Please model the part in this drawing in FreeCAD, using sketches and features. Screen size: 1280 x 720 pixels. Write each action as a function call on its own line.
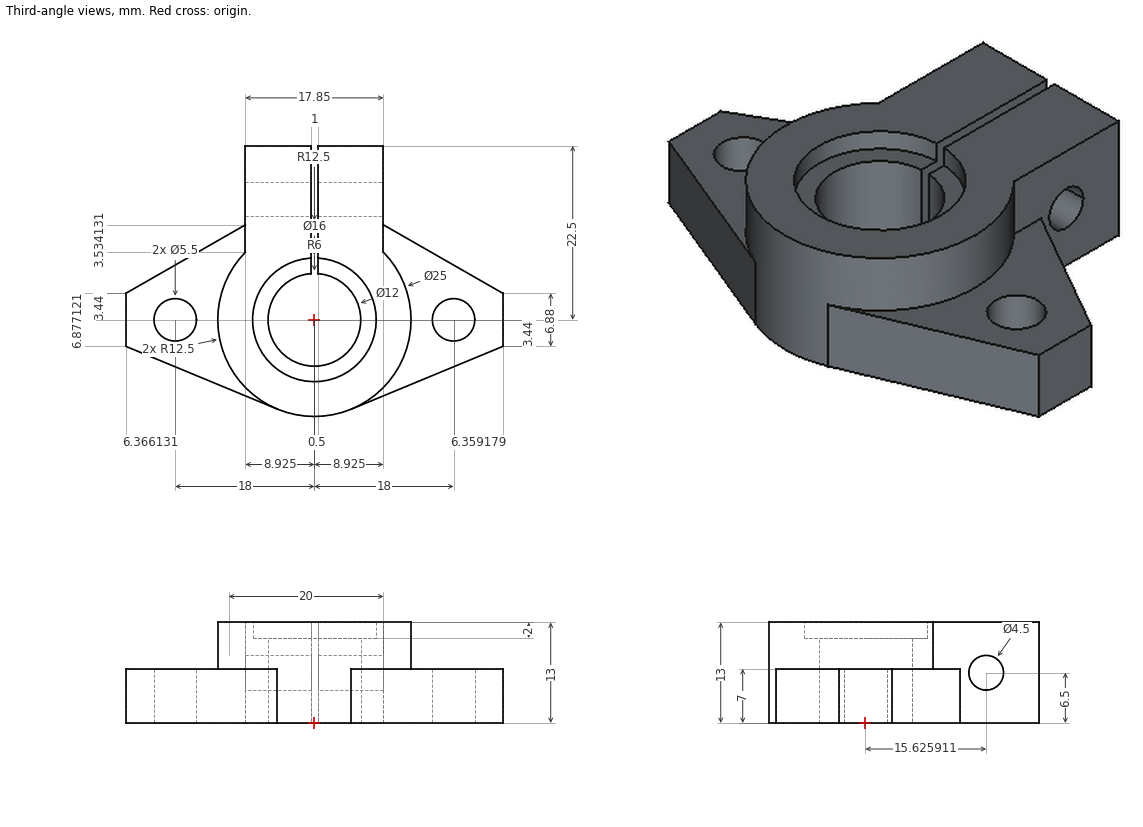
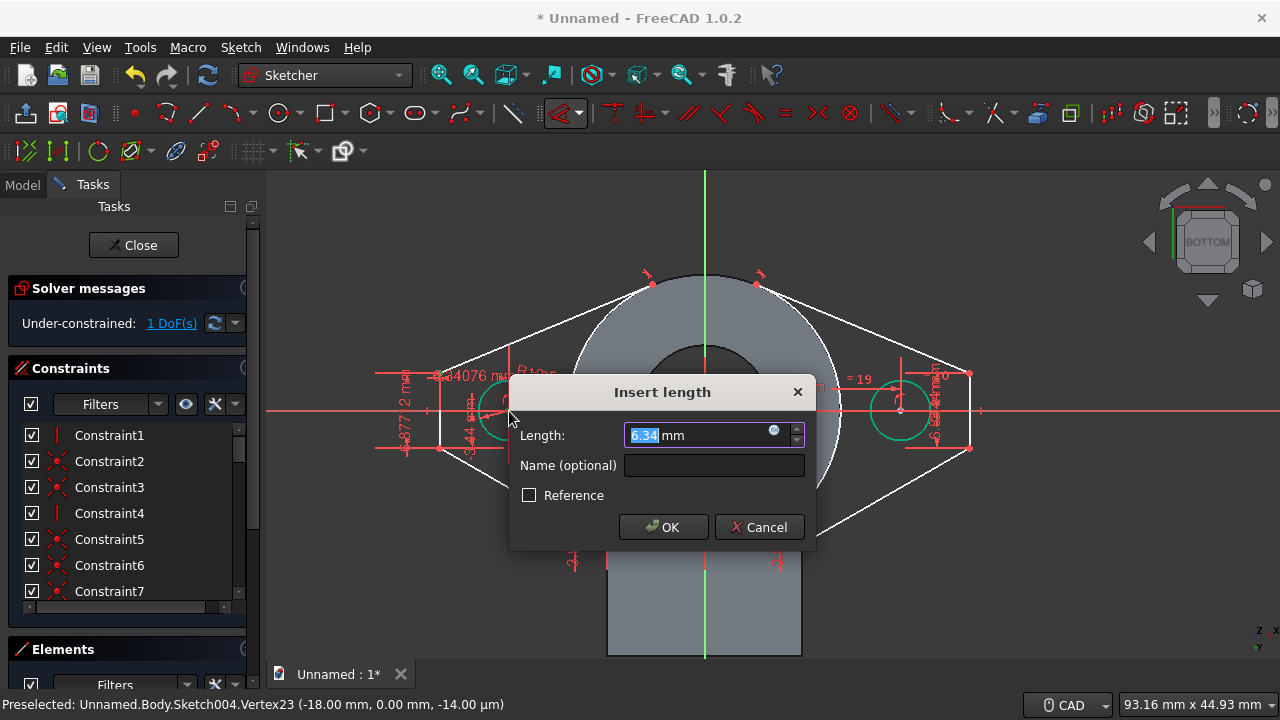
text(6.366131)
key(Return)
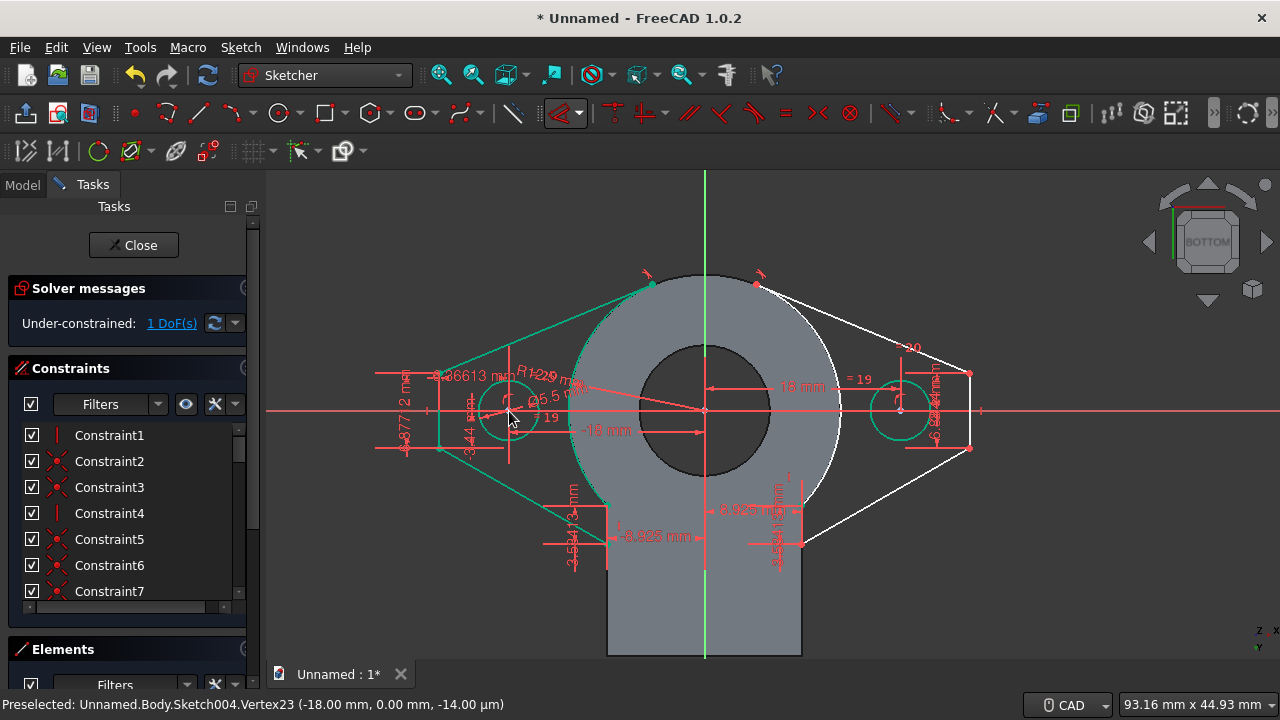
click(970, 373)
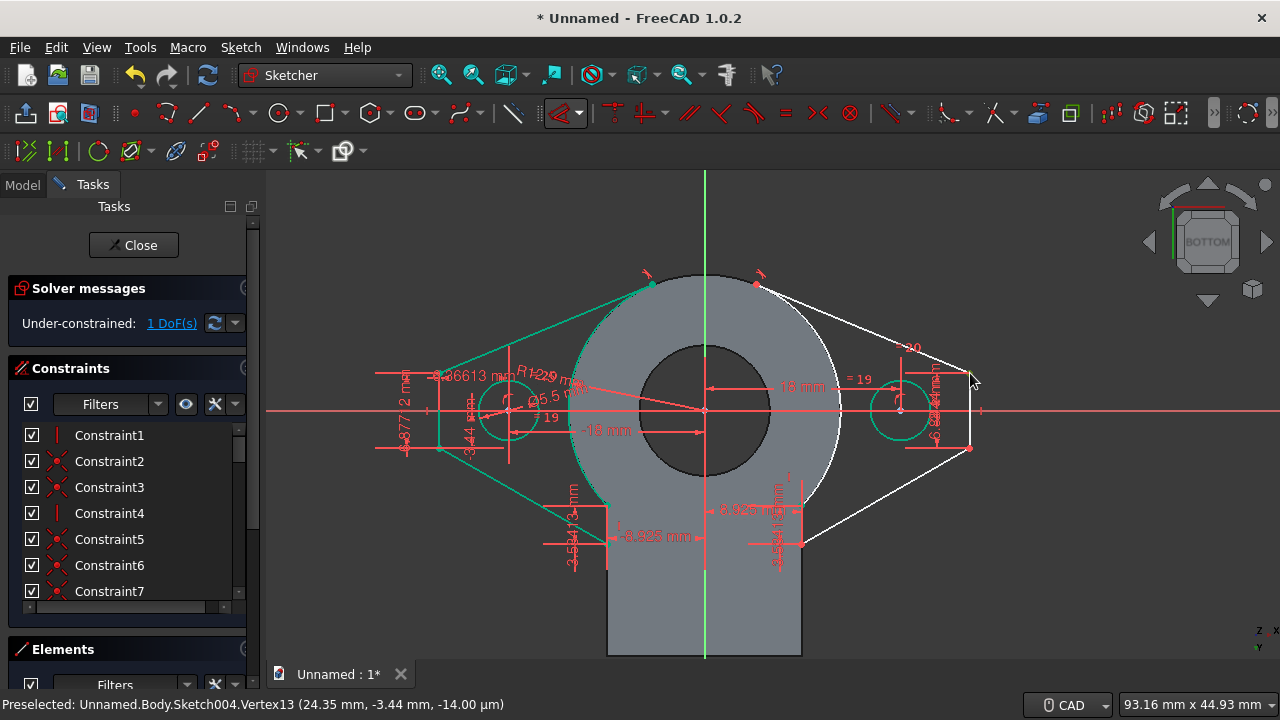
click(901, 411)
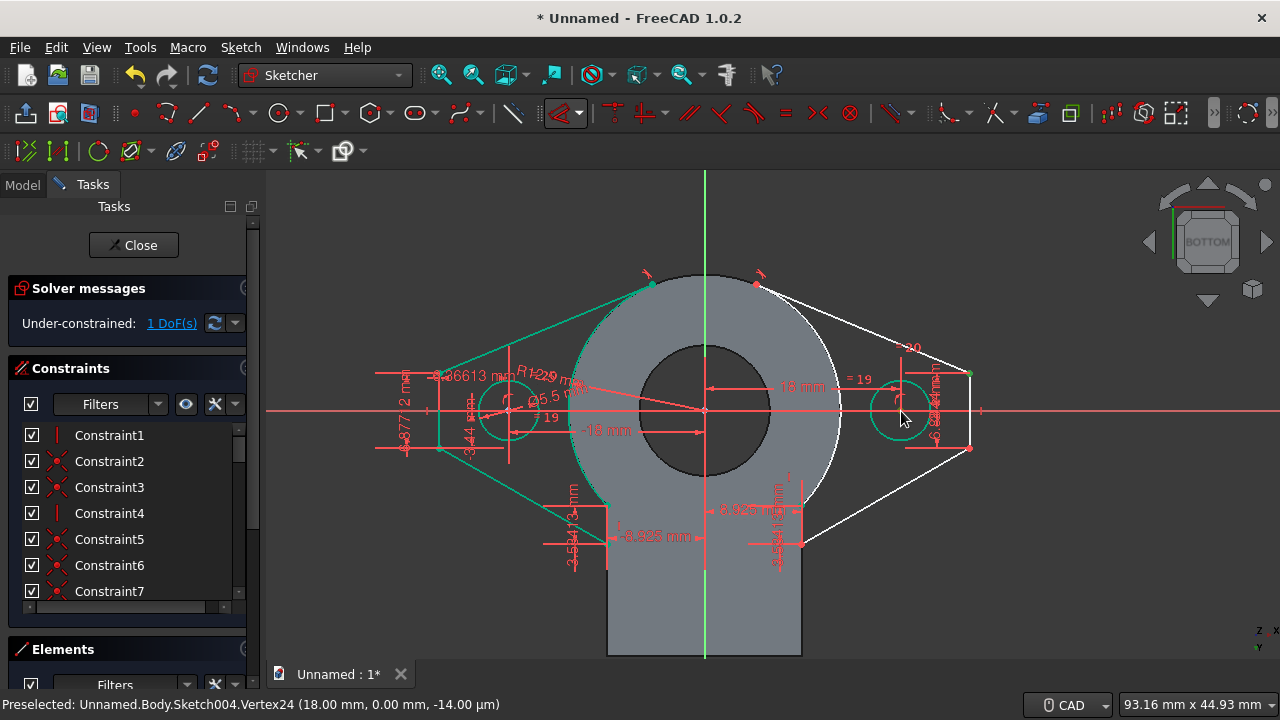
click(582, 114)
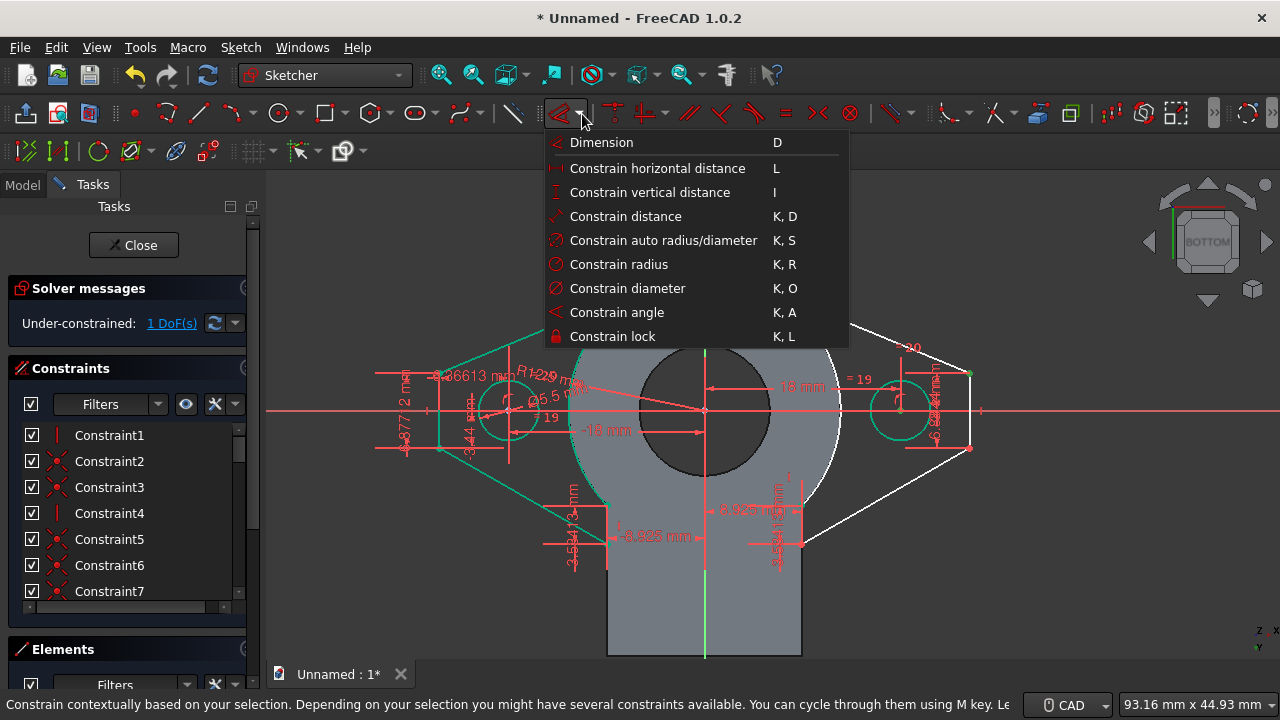
click(697, 168)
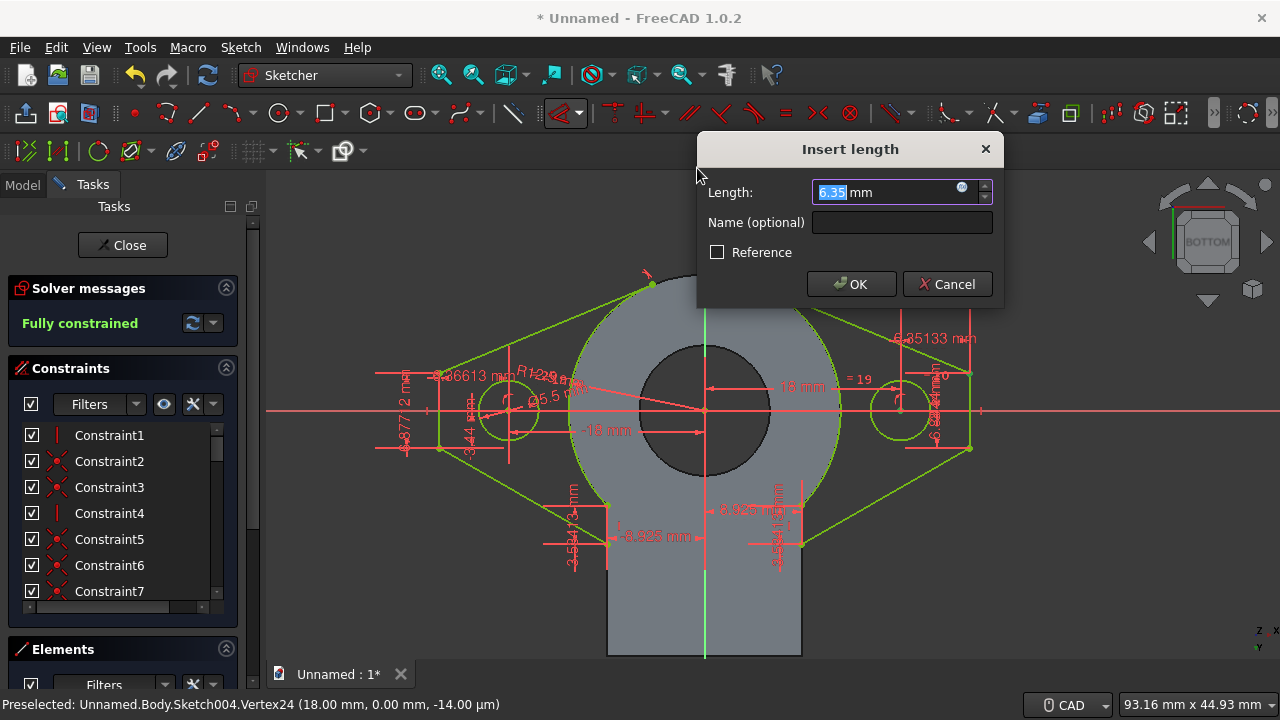
text(6.359179)
key(Return)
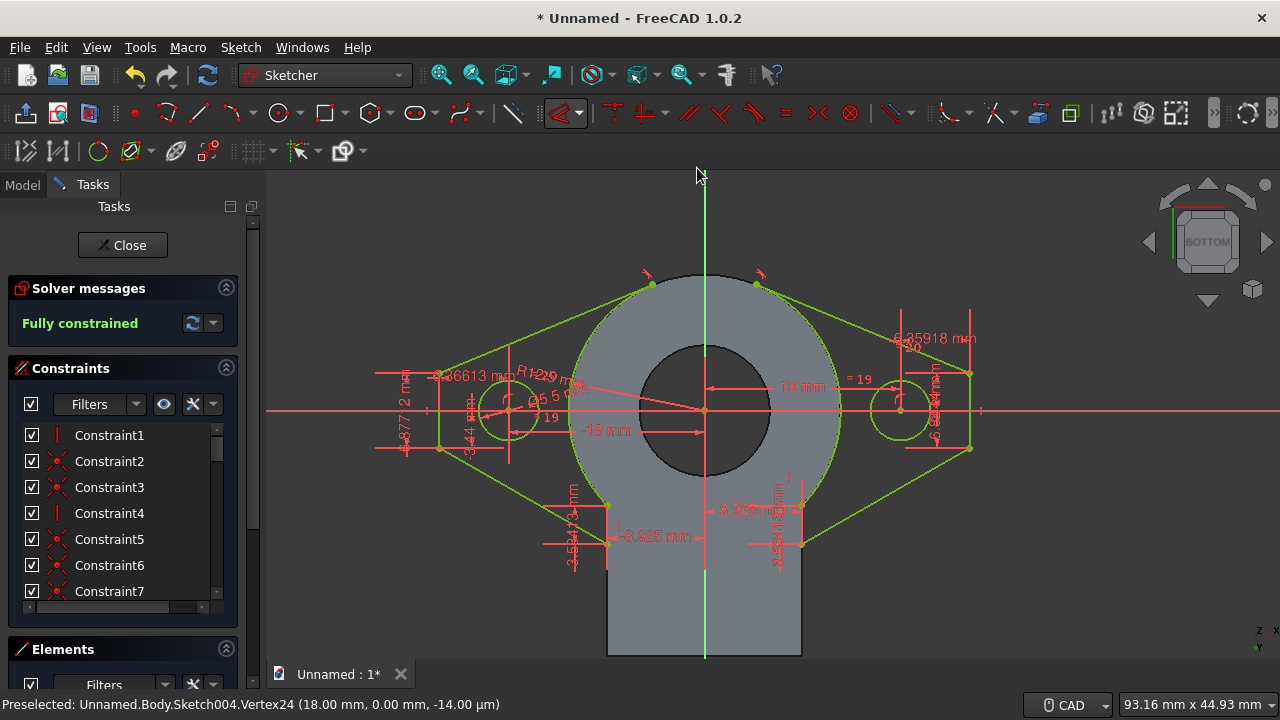
click(123, 245)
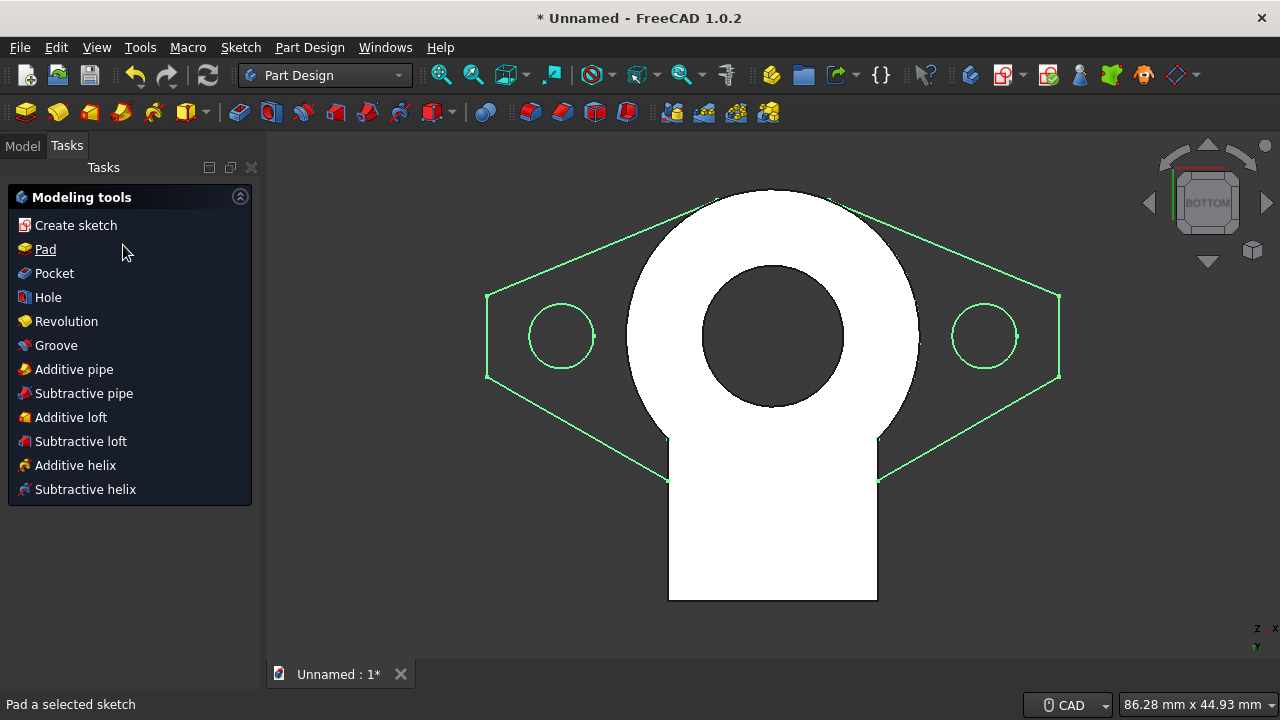
click(26, 112)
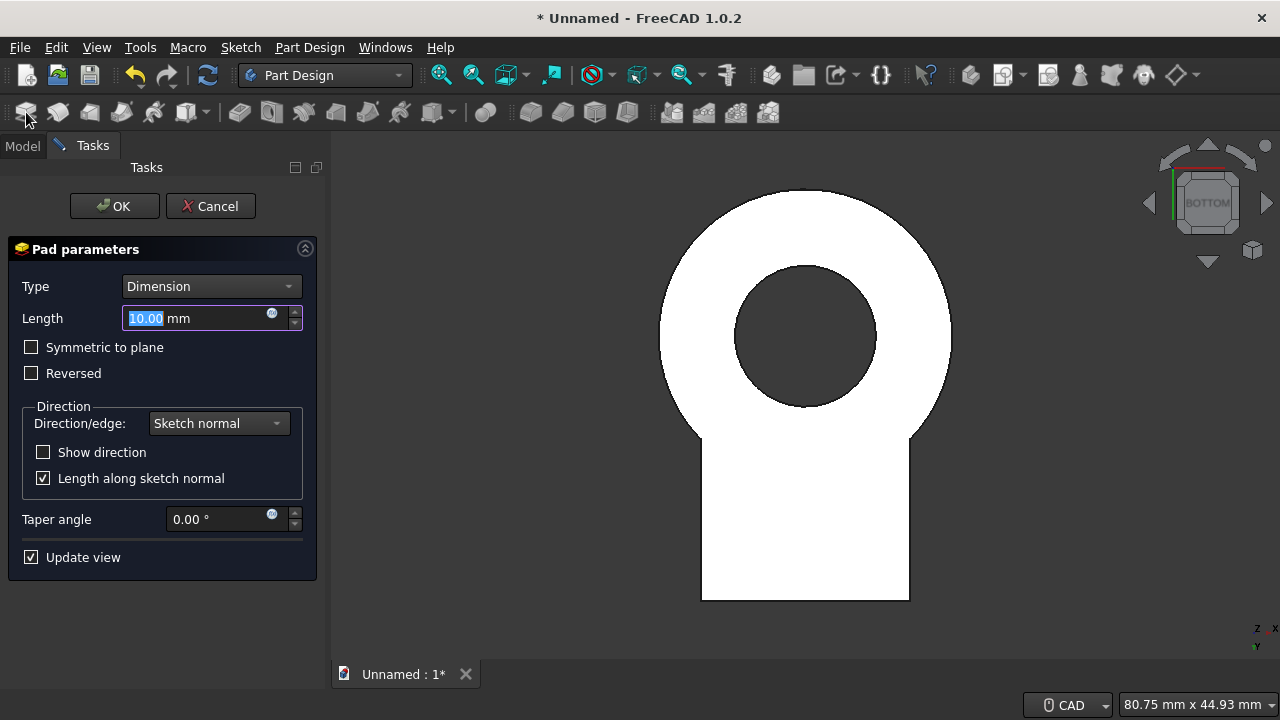
text(7)
key(Tab)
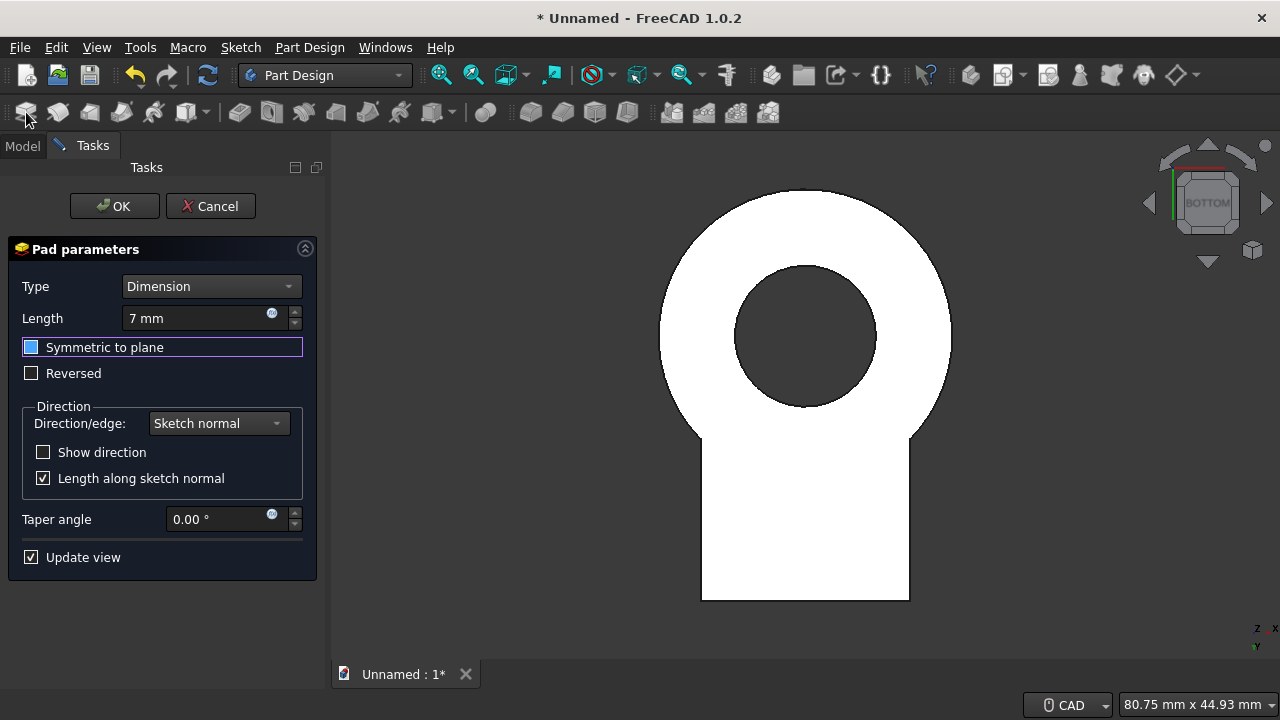
click(30, 373)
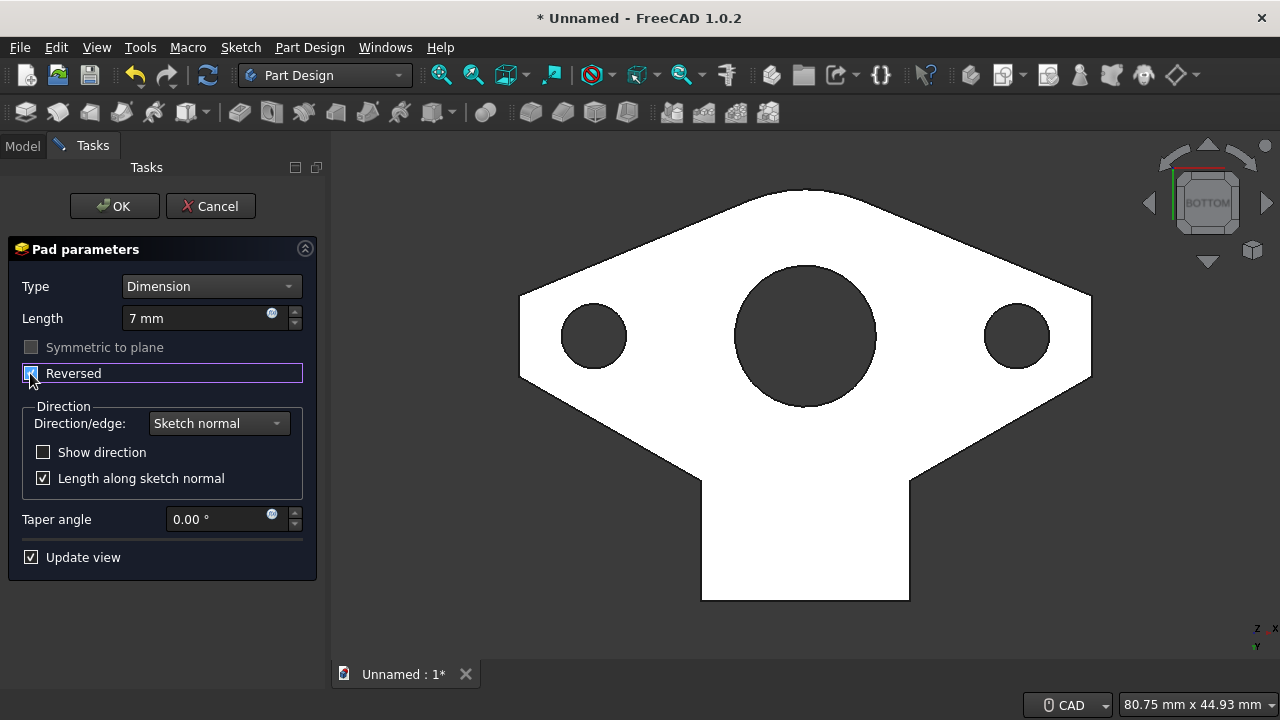
click(115, 206)